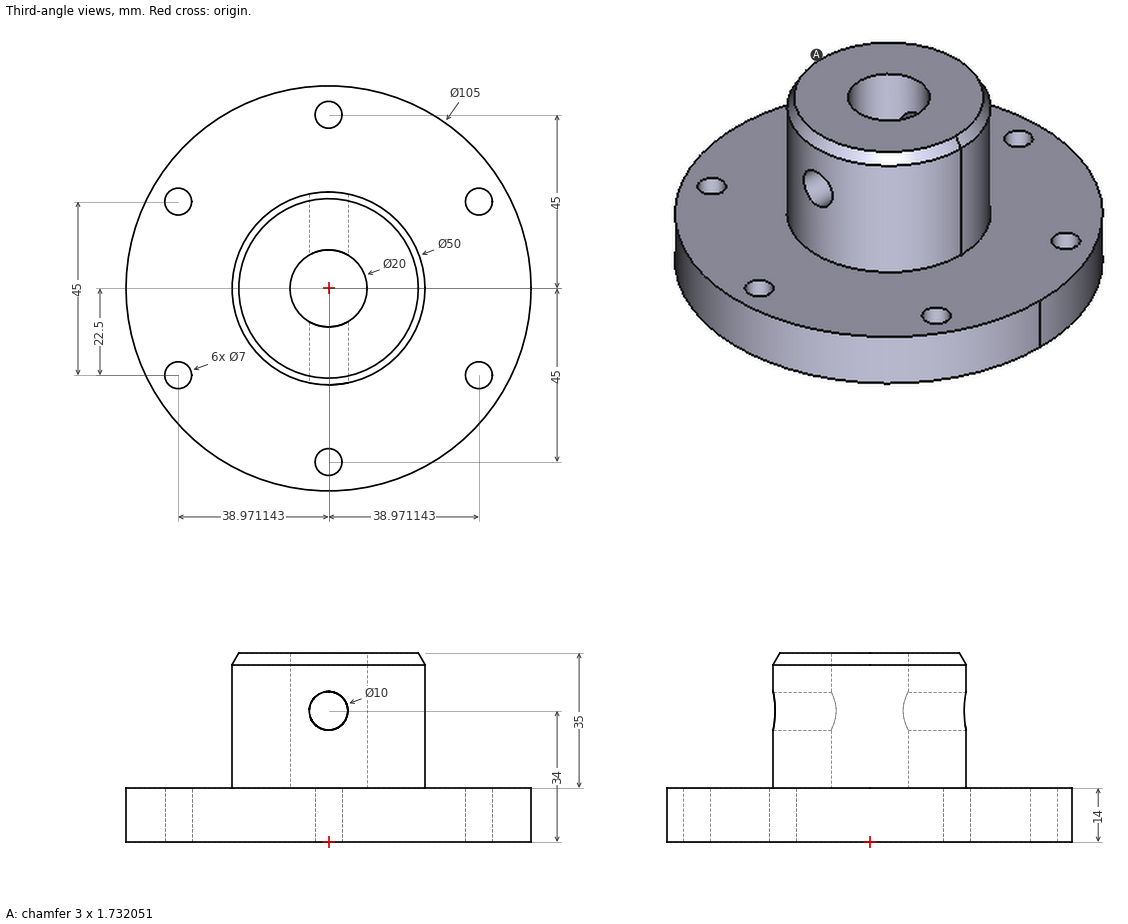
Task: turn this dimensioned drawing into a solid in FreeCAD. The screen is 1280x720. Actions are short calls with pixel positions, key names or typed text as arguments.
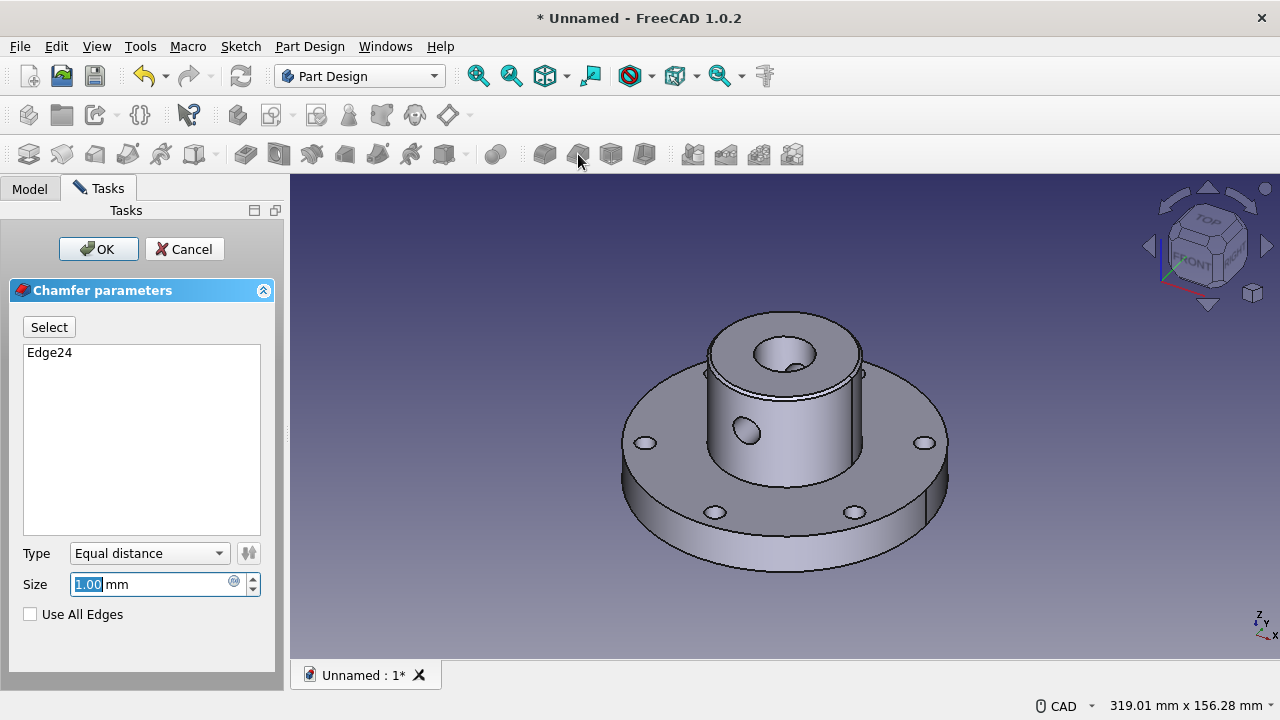
text(3)
key(Tab)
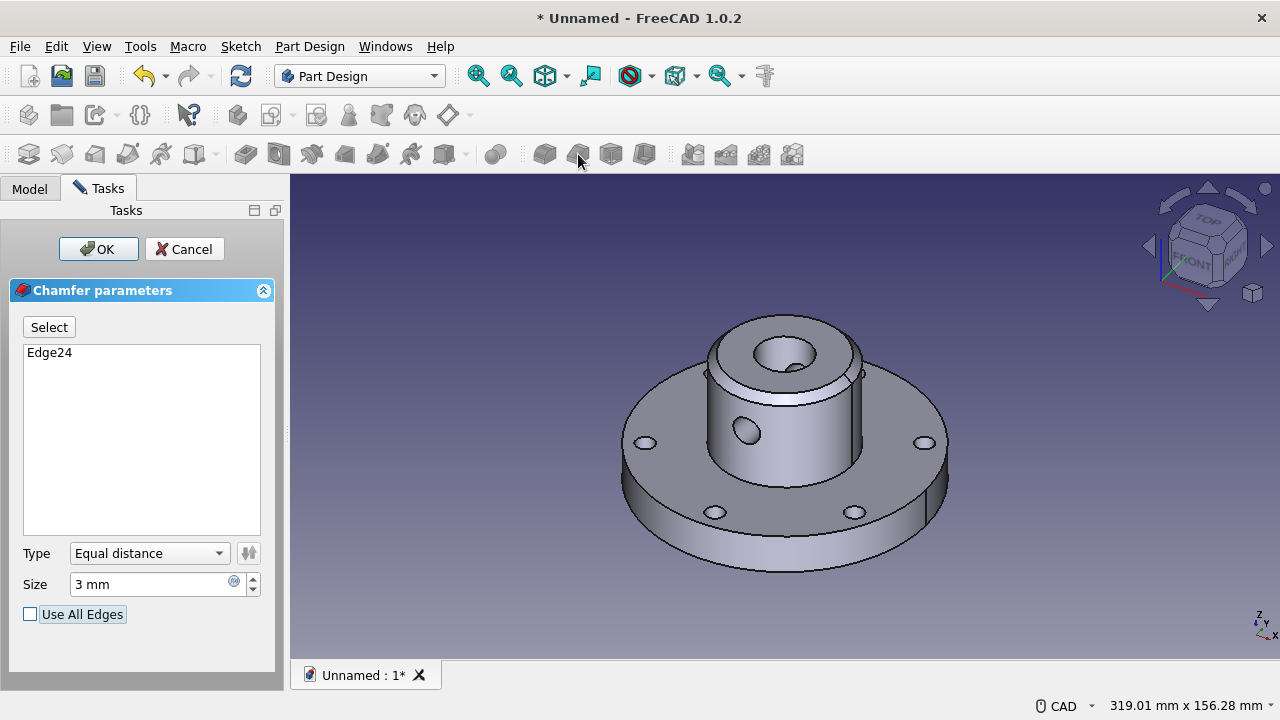
click(150, 554)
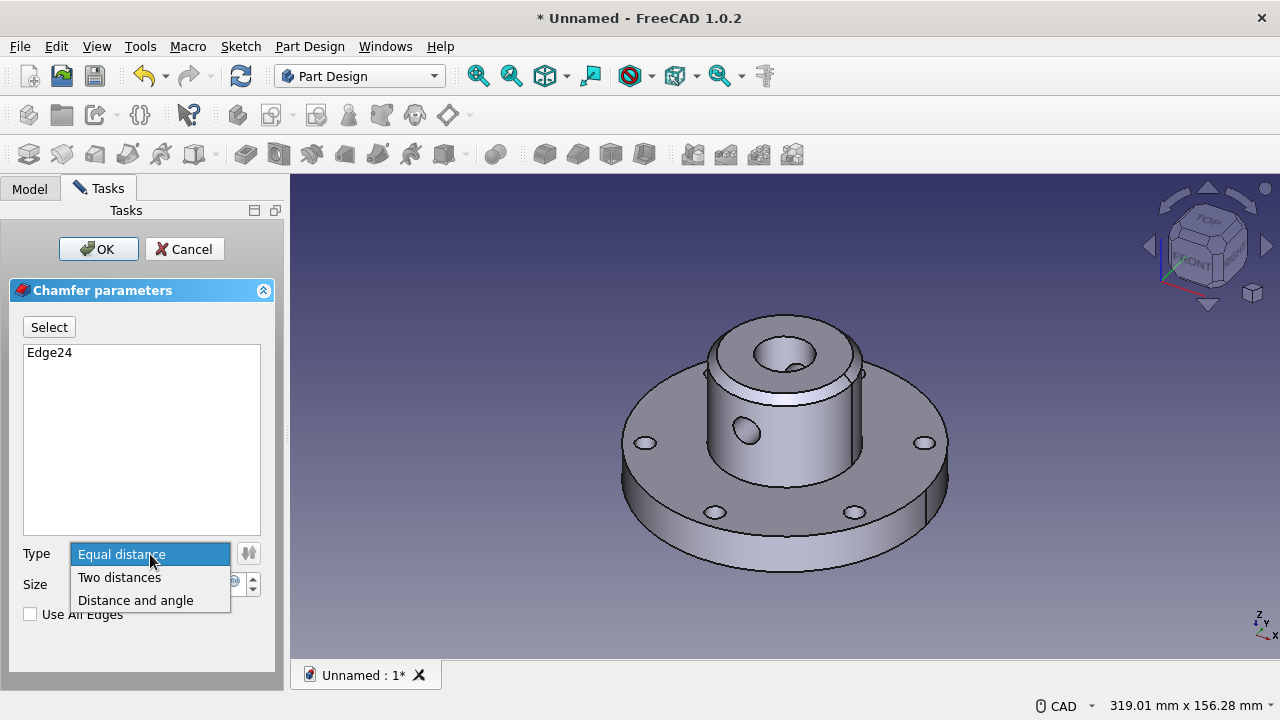
click(148, 578)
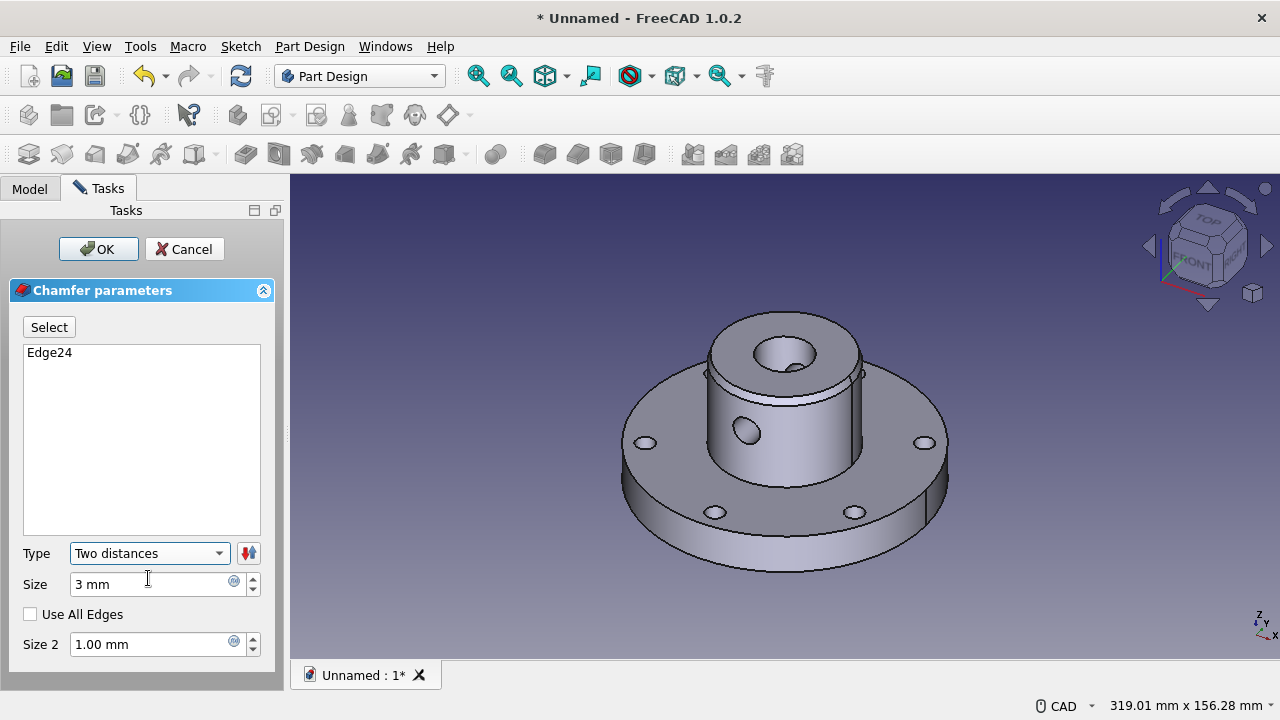
triple_click(158, 644)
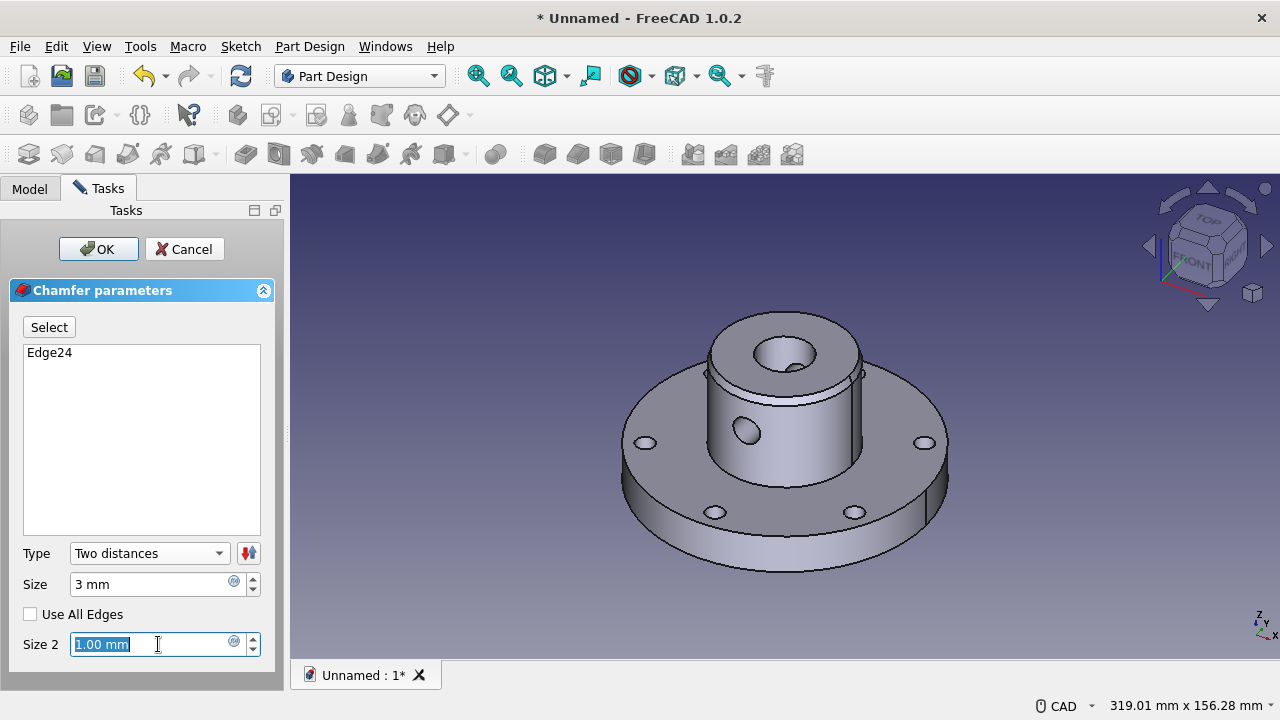
text(1.732051)
key(Tab)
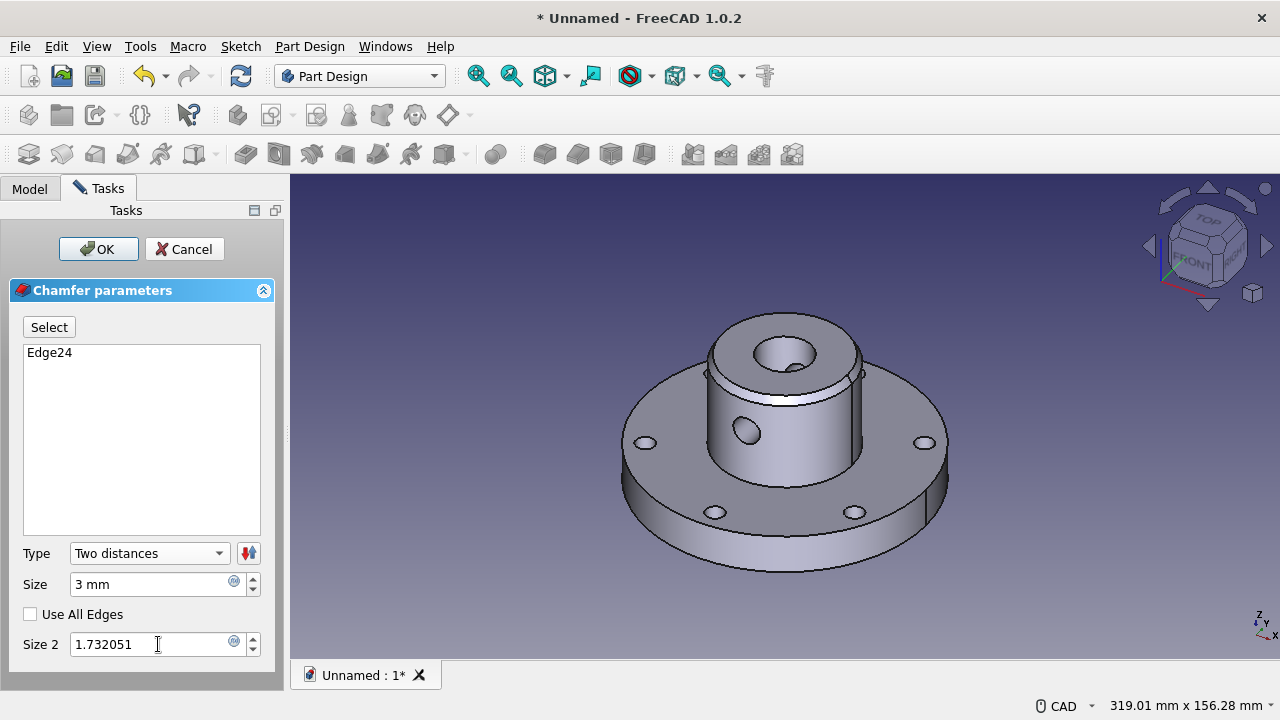
click(99, 249)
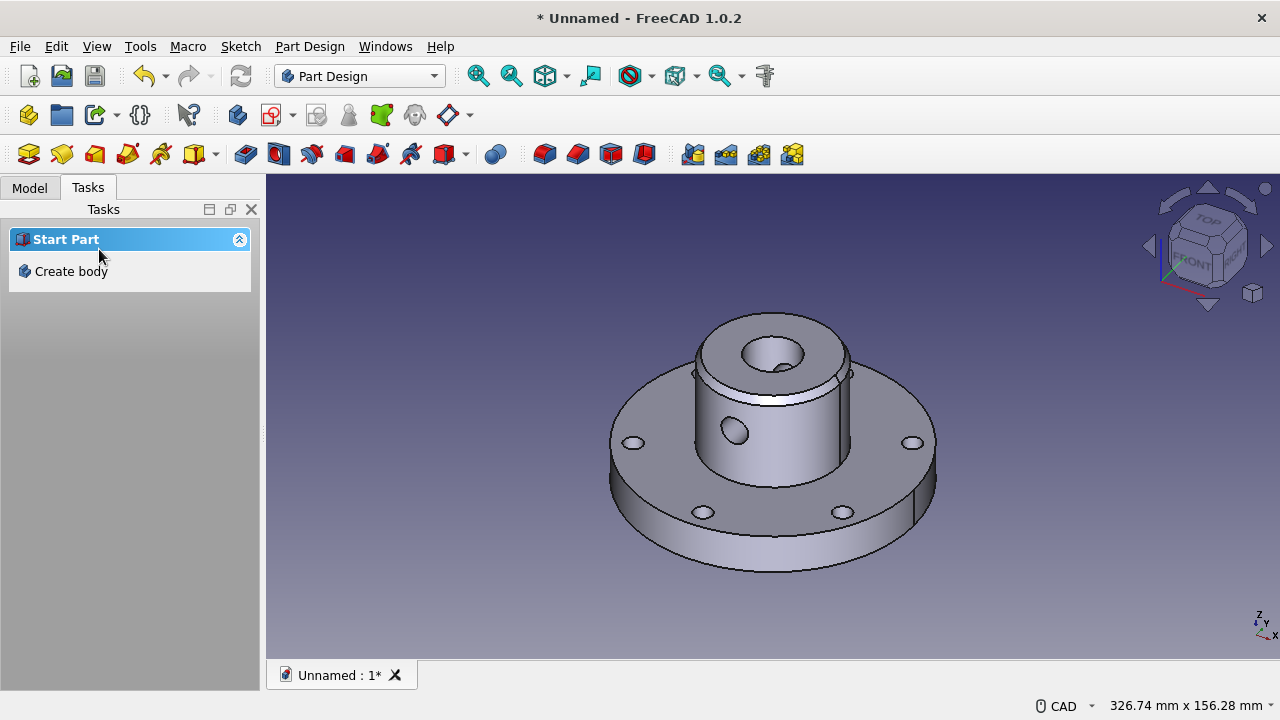
key(0)